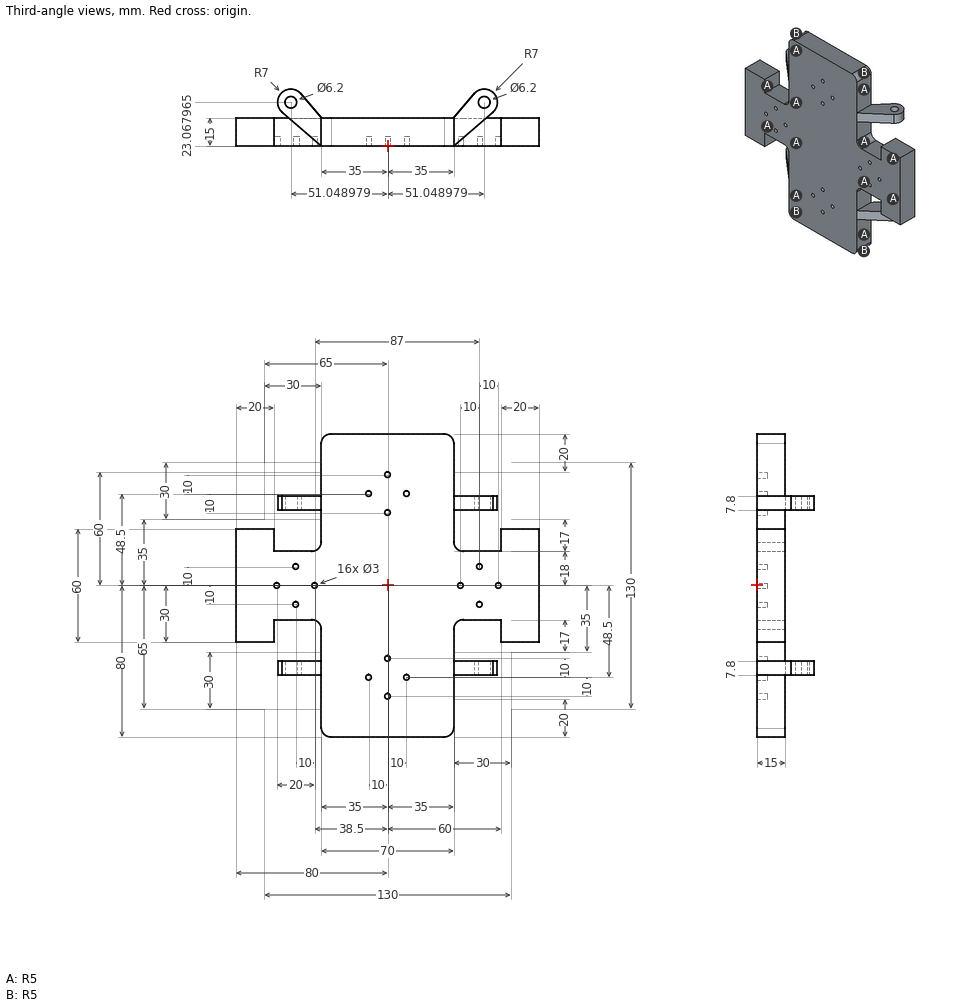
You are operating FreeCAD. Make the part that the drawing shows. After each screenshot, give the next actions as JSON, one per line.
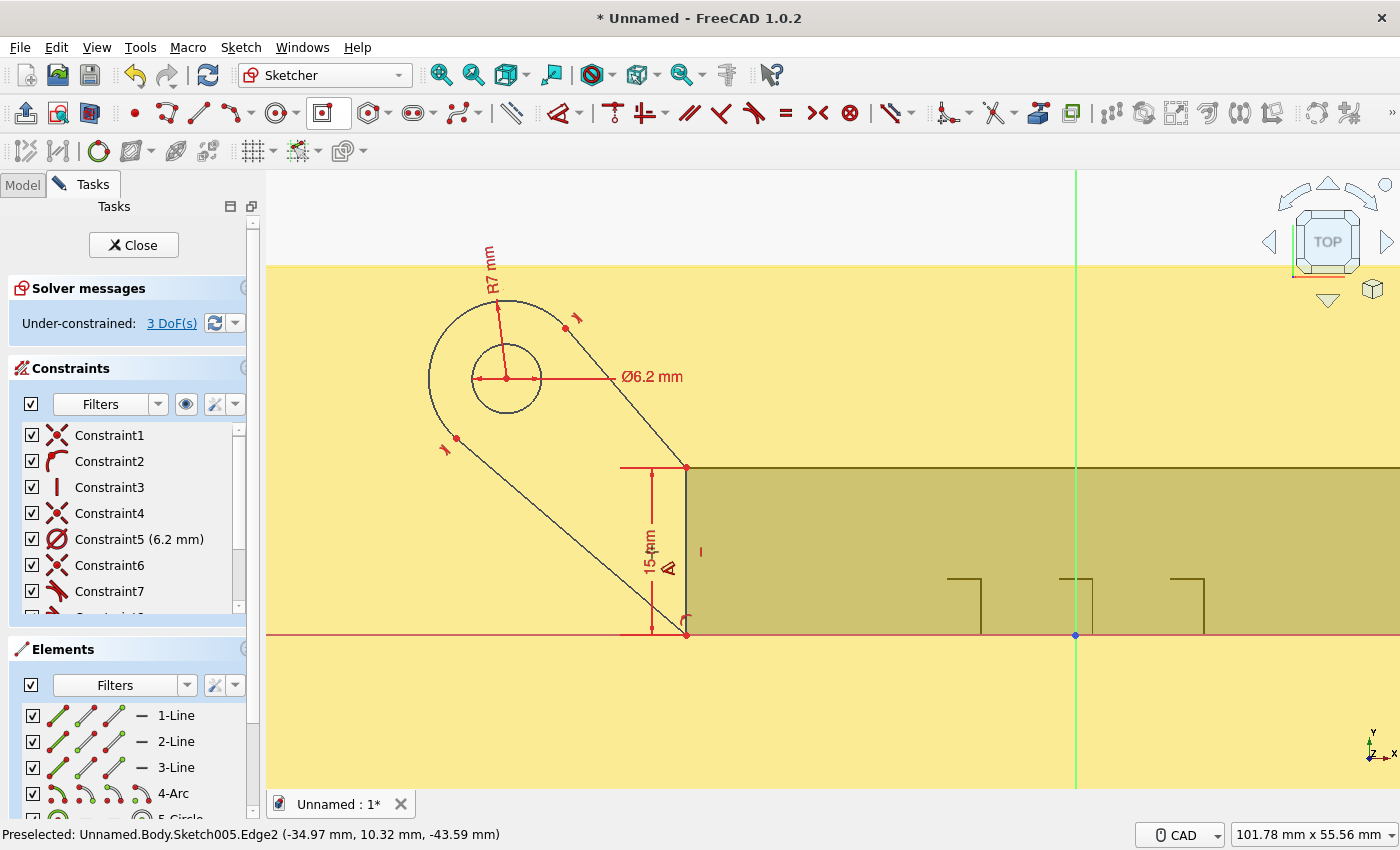
{"action": "left_click", "coordinate": [686, 468]}
{"action": "left_click", "coordinate": [881, 669]}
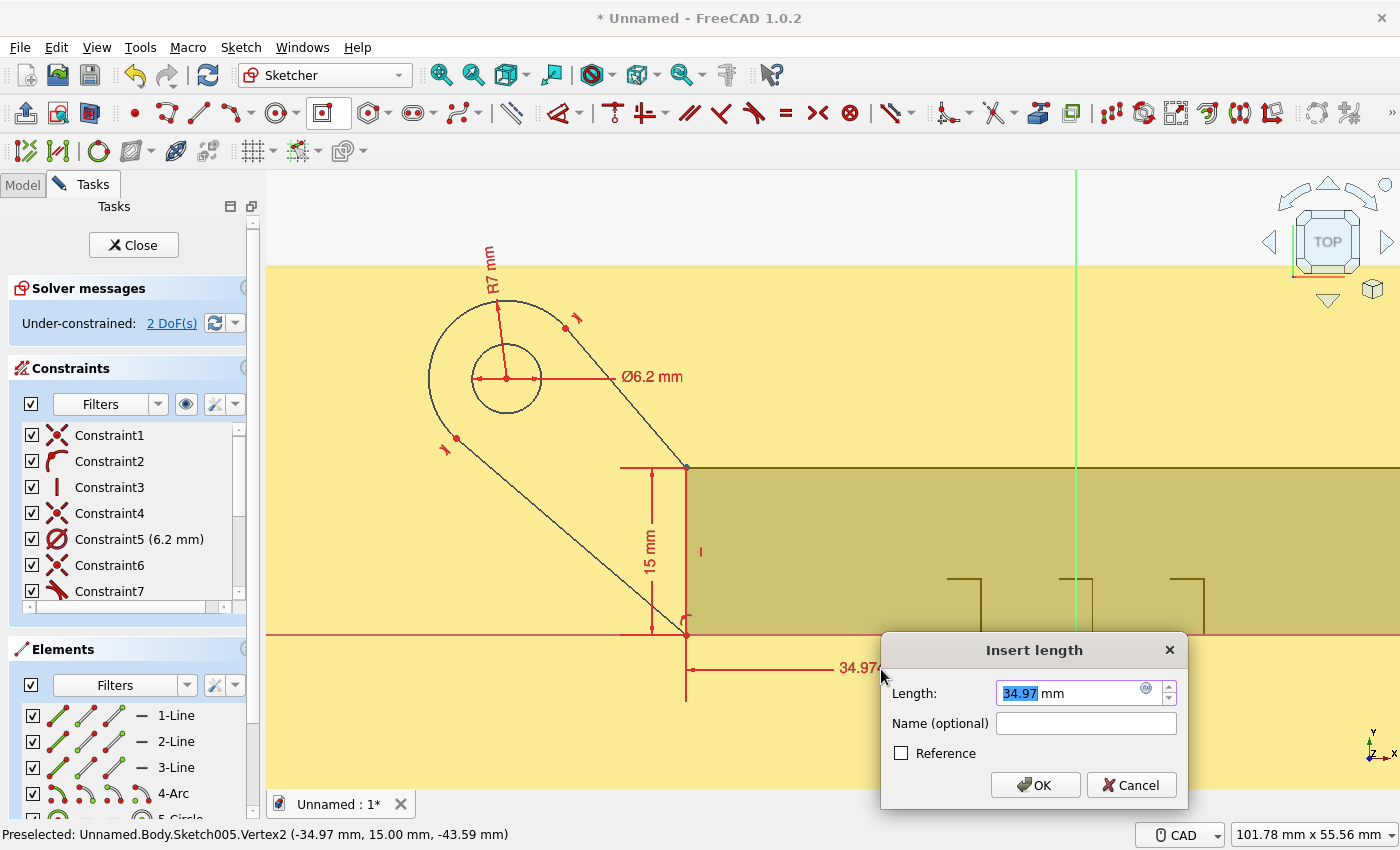
{"action": "type", "text": "35"}
{"action": "key", "text": "Return"}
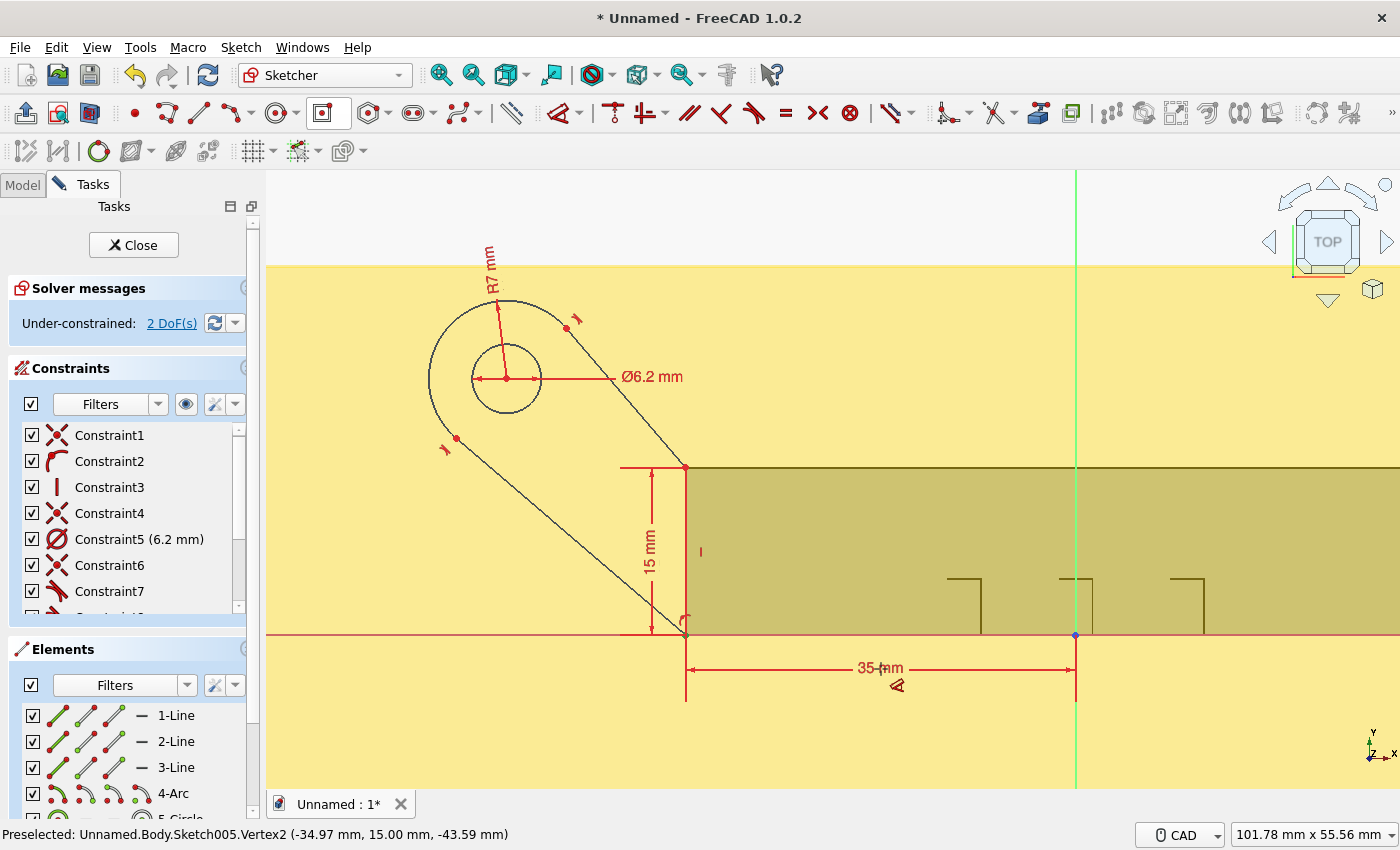
{"action": "left_click", "coordinate": [507, 379]}
{"action": "left_click", "coordinate": [791, 669]}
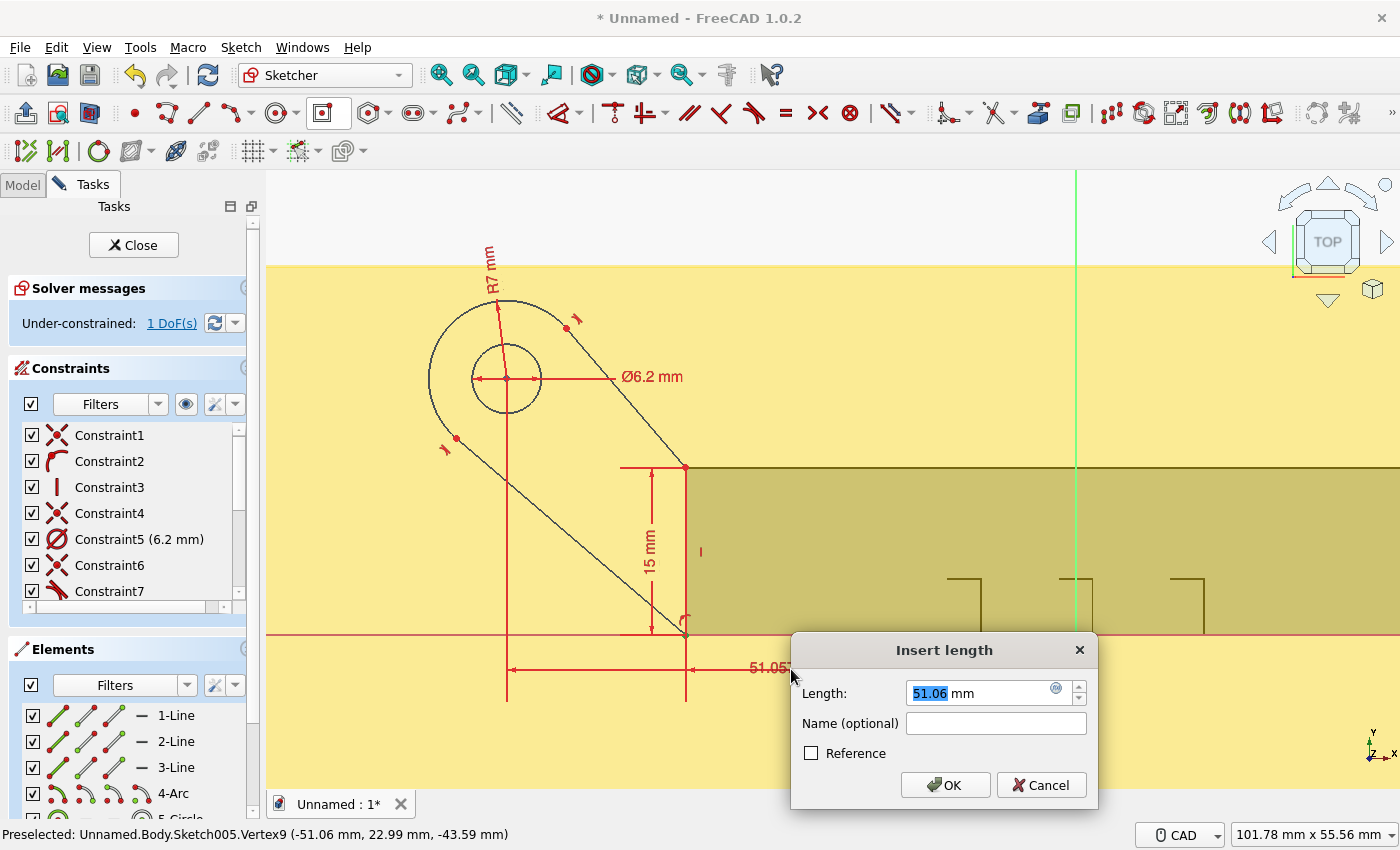
{"action": "type", "text": "51.048979"}
{"action": "key", "text": "Return"}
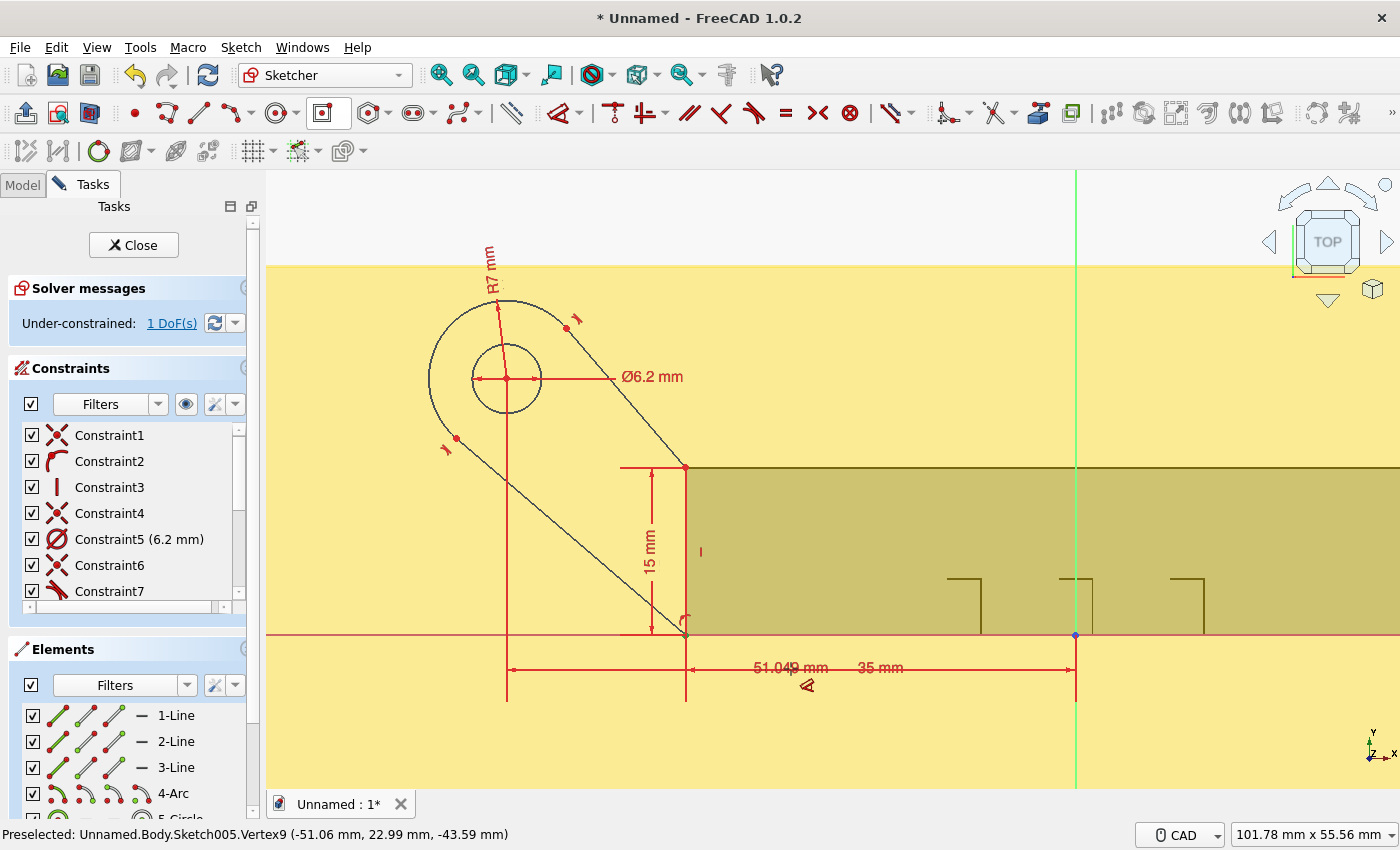
{"action": "left_click", "coordinate": [507, 379]}
{"action": "left_click", "coordinate": [1110, 507]}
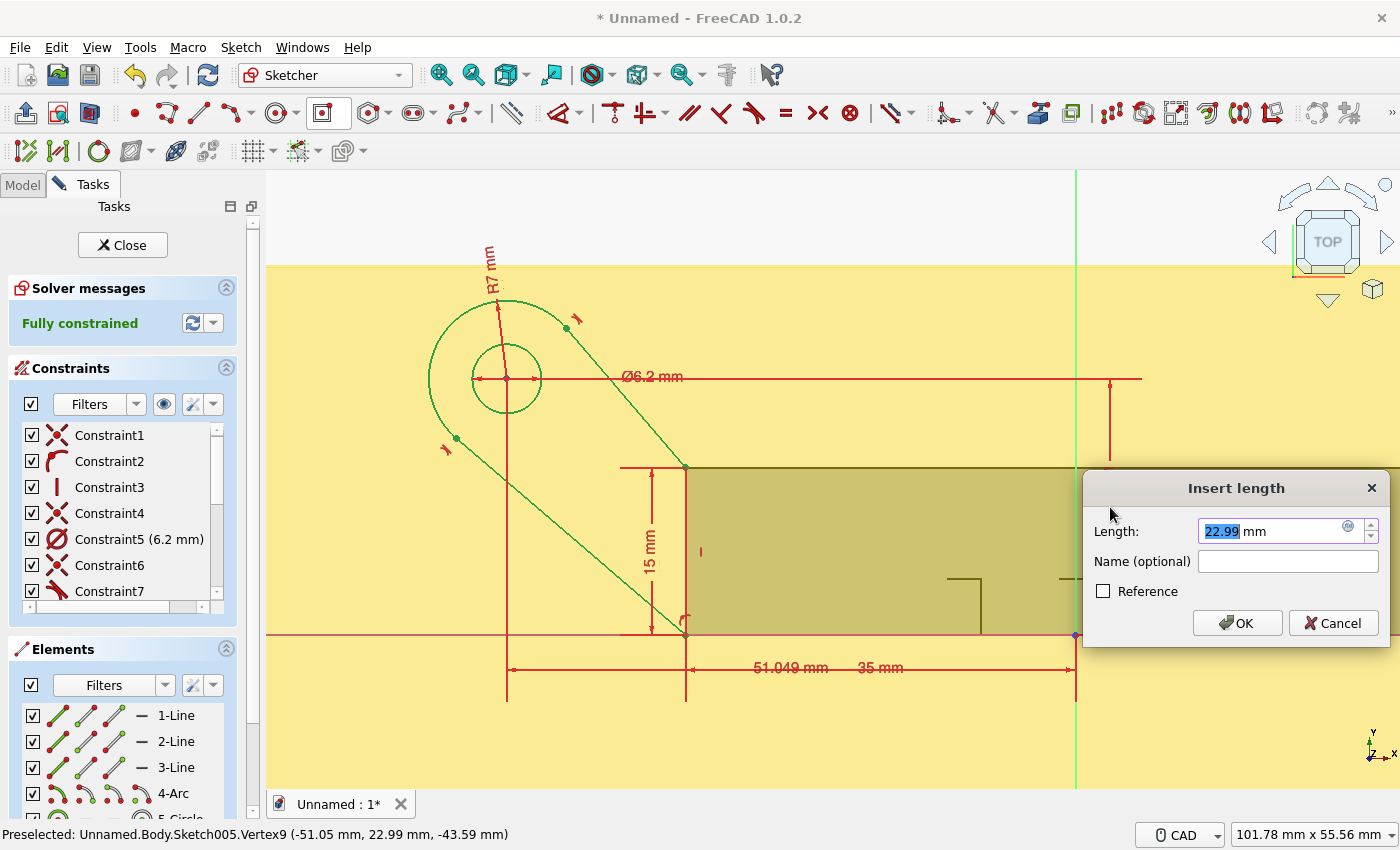
{"action": "type", "text": "23.067965"}
{"action": "key", "text": "Return"}
{"action": "key", "text": "Escape"}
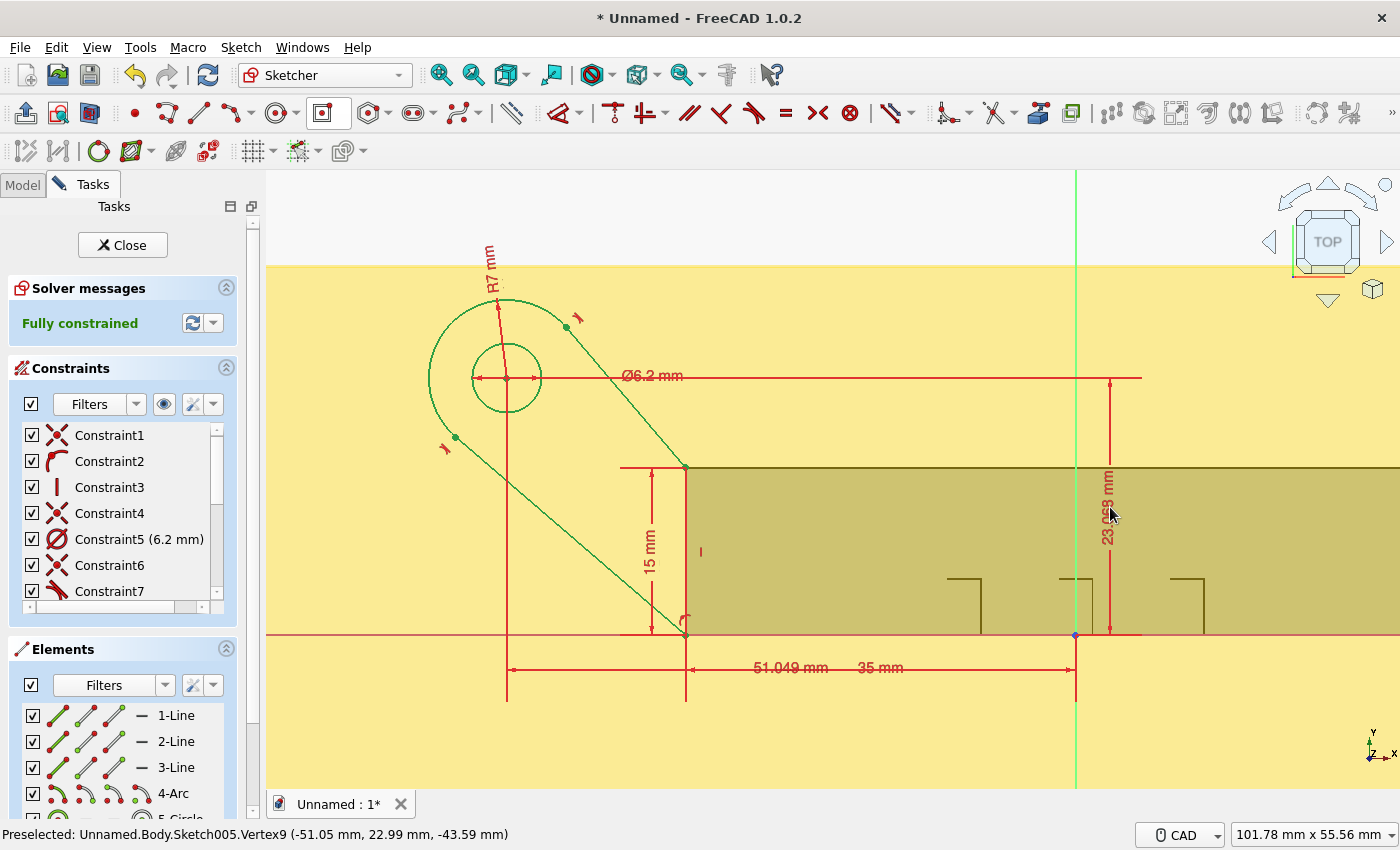
{"action": "left_click", "coordinate": [123, 245]}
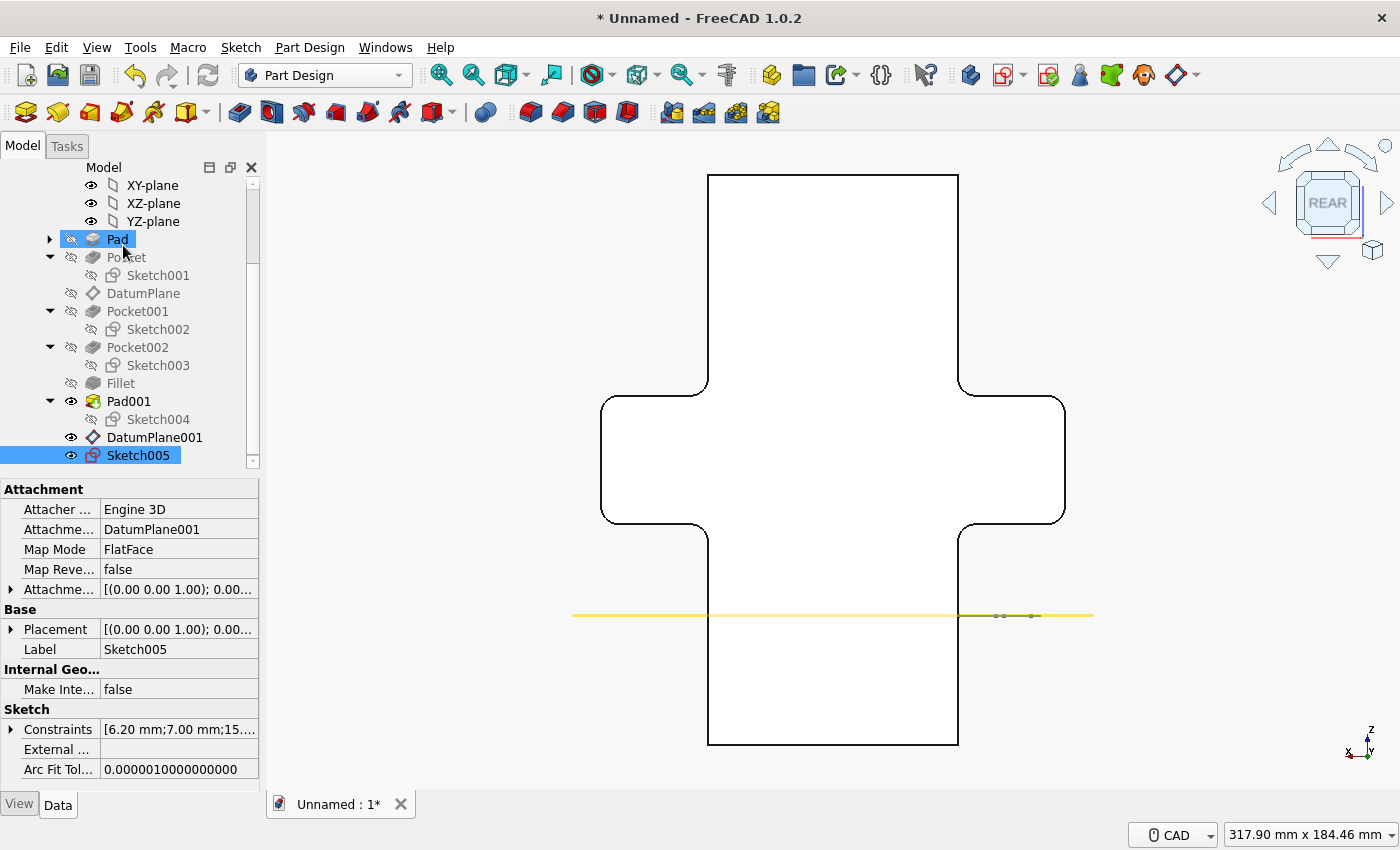
{"action": "left_click", "coordinate": [26, 112]}